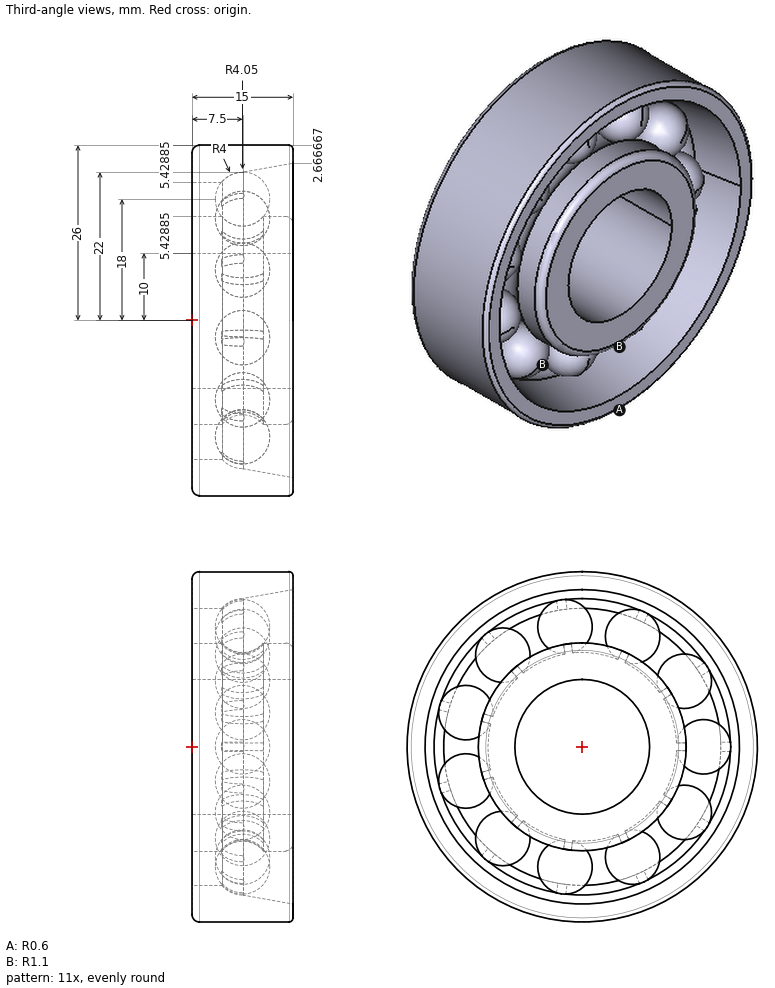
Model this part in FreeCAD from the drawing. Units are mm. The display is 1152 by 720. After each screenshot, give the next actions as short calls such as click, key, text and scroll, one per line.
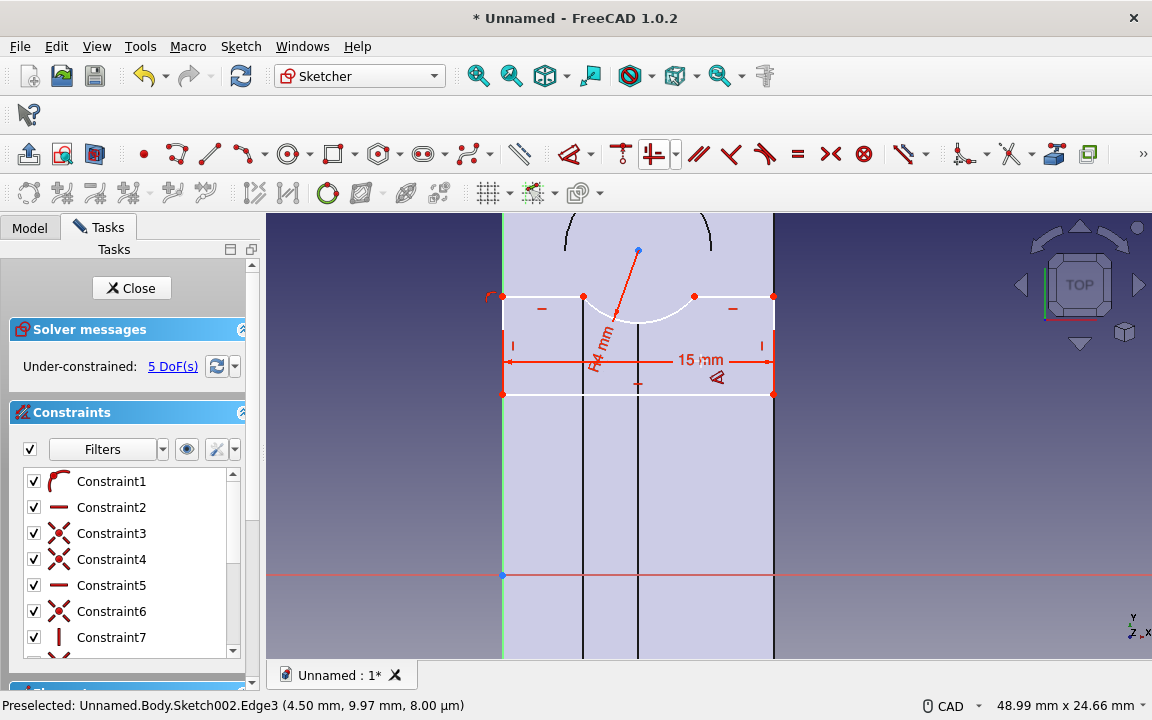
click(503, 395)
click(469, 485)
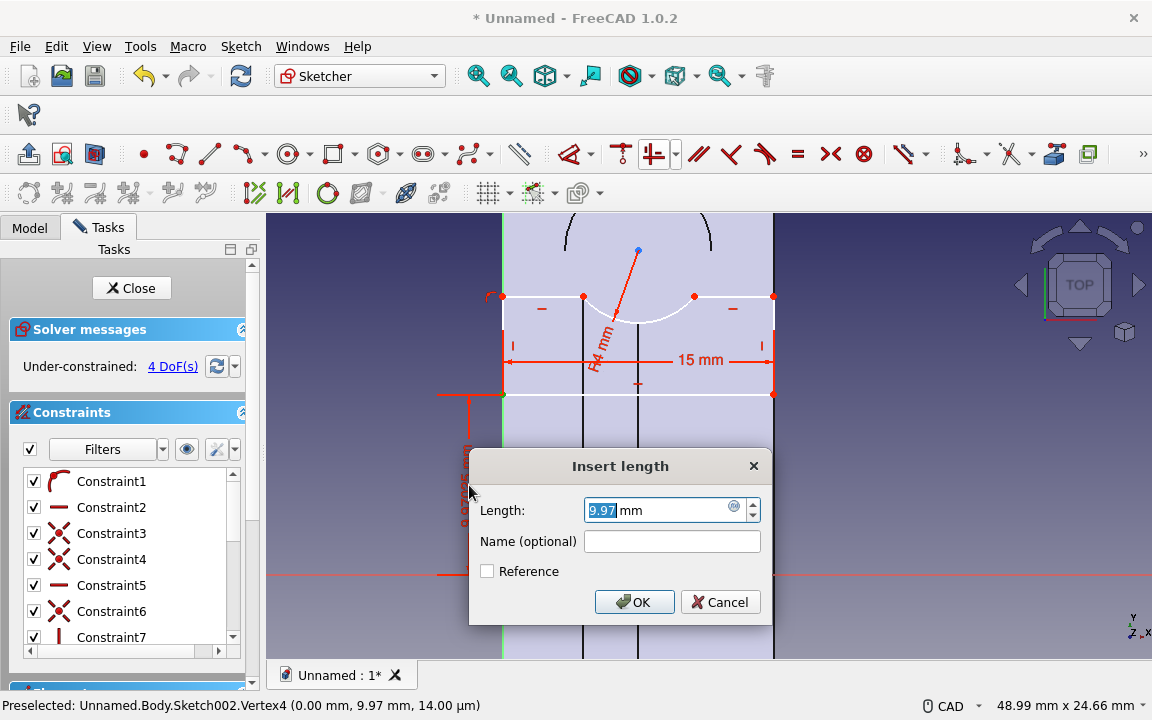
text(10)
key(Return)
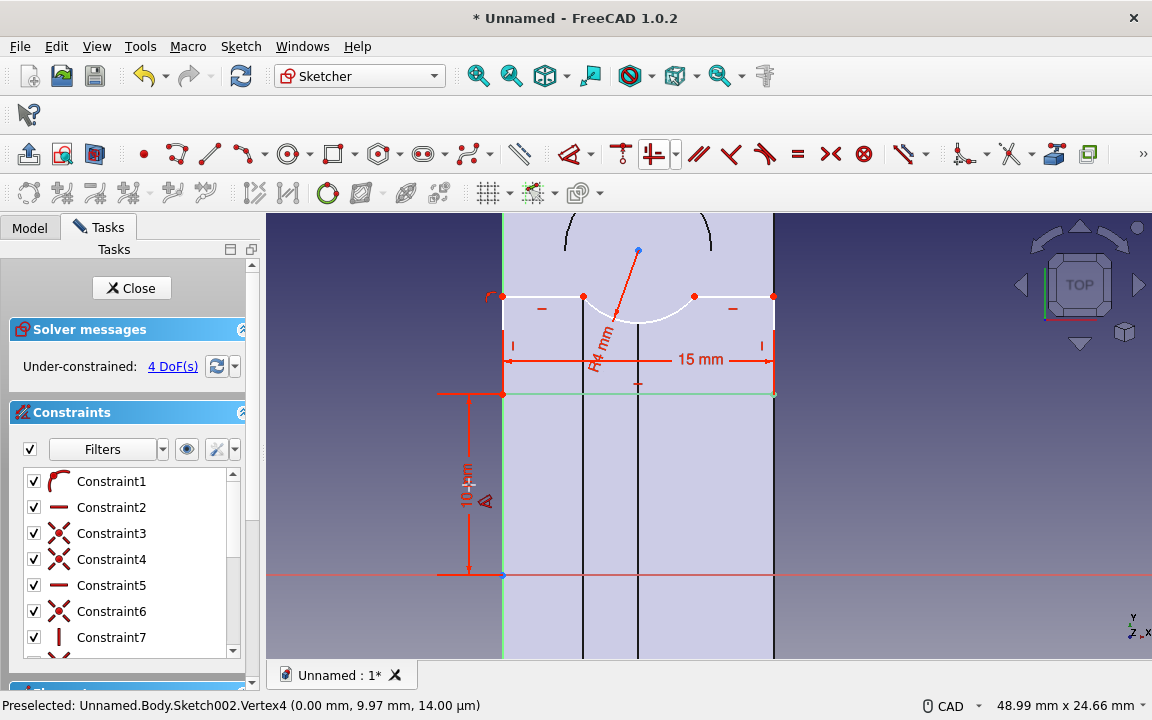
click(638, 251)
click(469, 413)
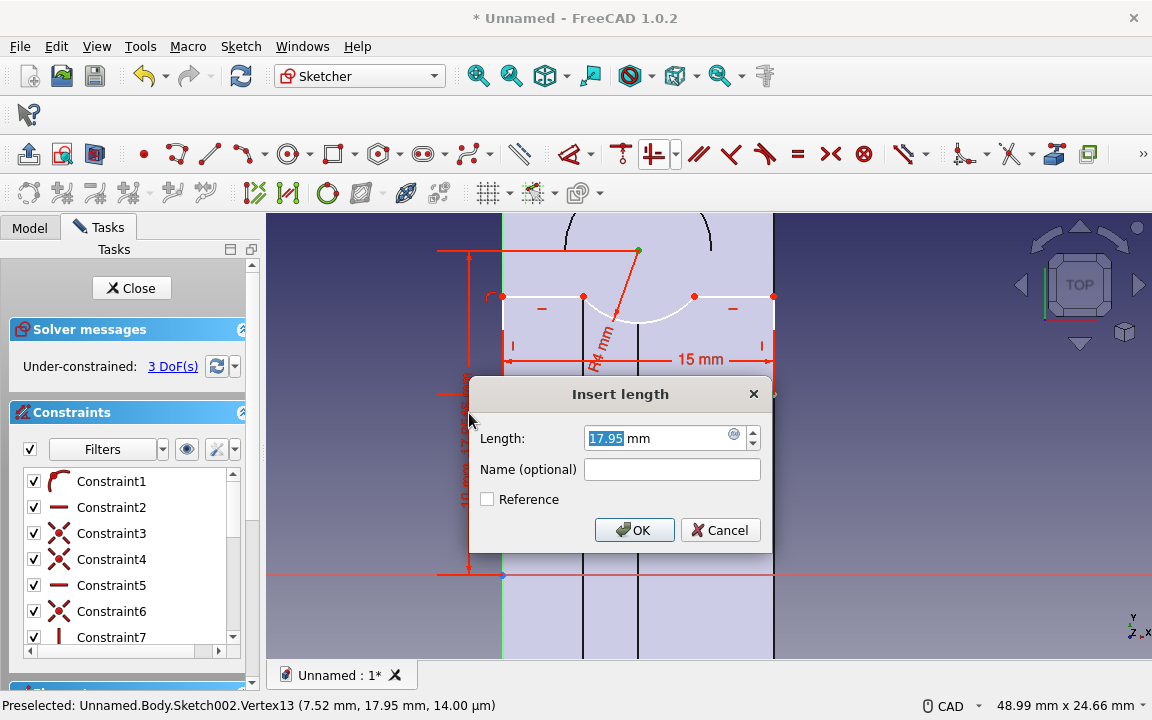
text(18)
key(Return)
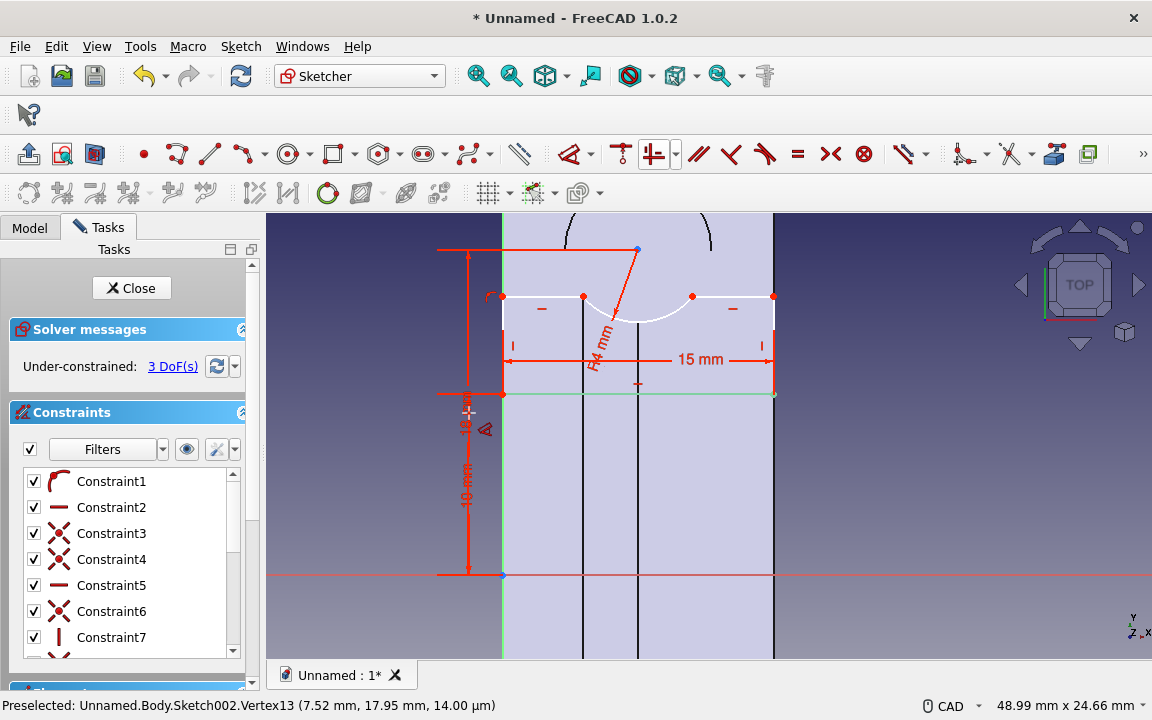
click(638, 250)
click(570, 609)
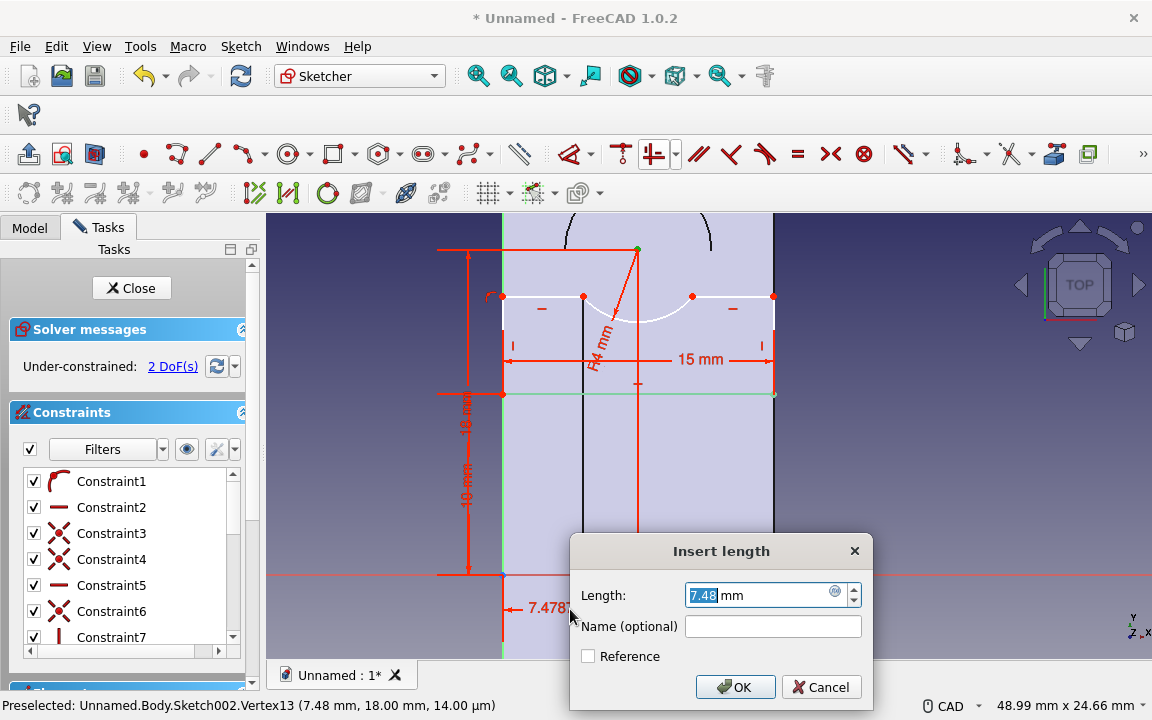
text(7.5)
key(Return)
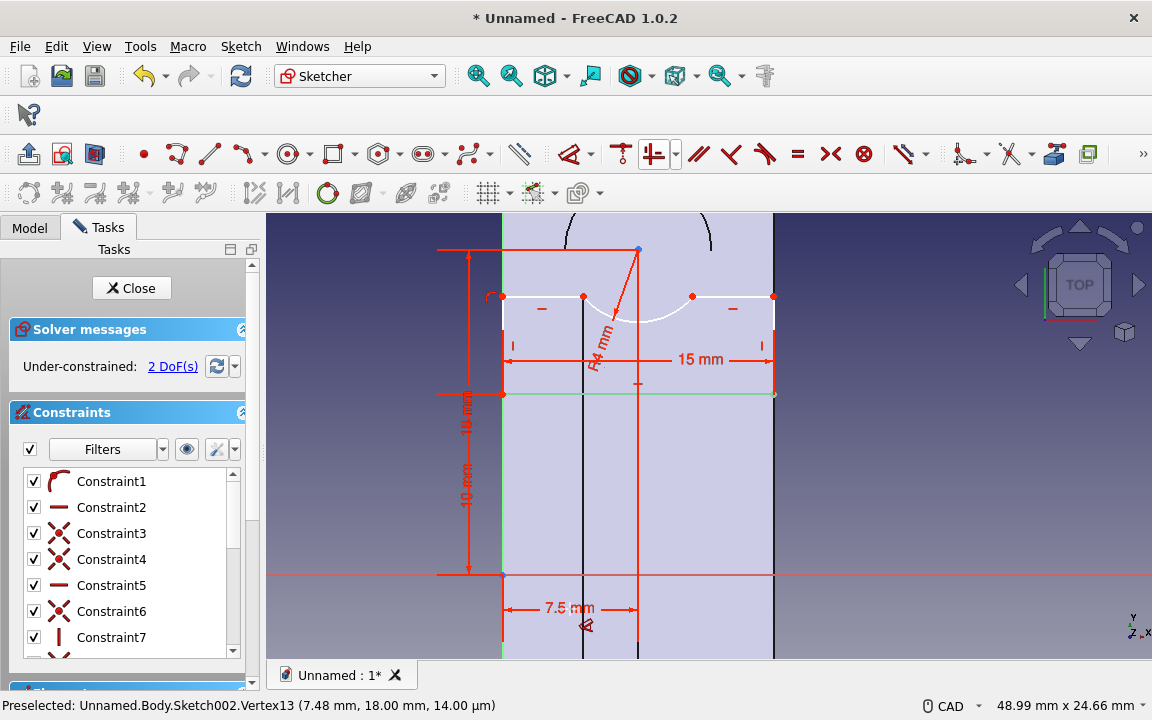
click(503, 326)
click(469, 346)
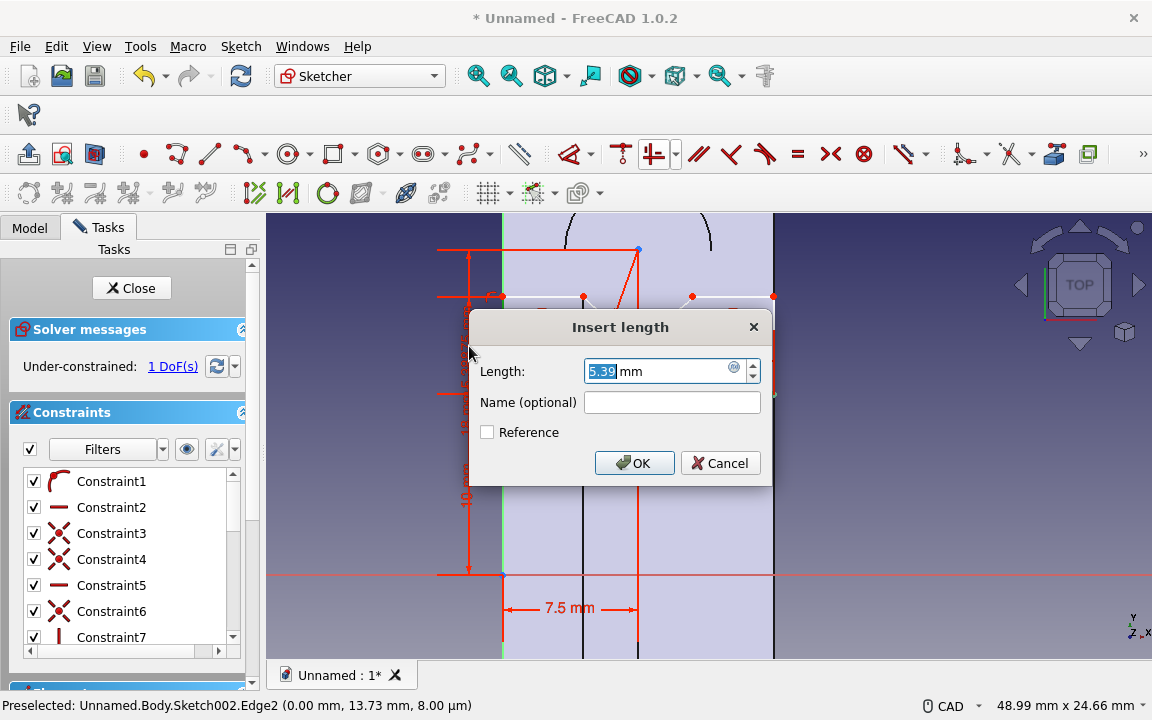
text(5.42885)
key(Return)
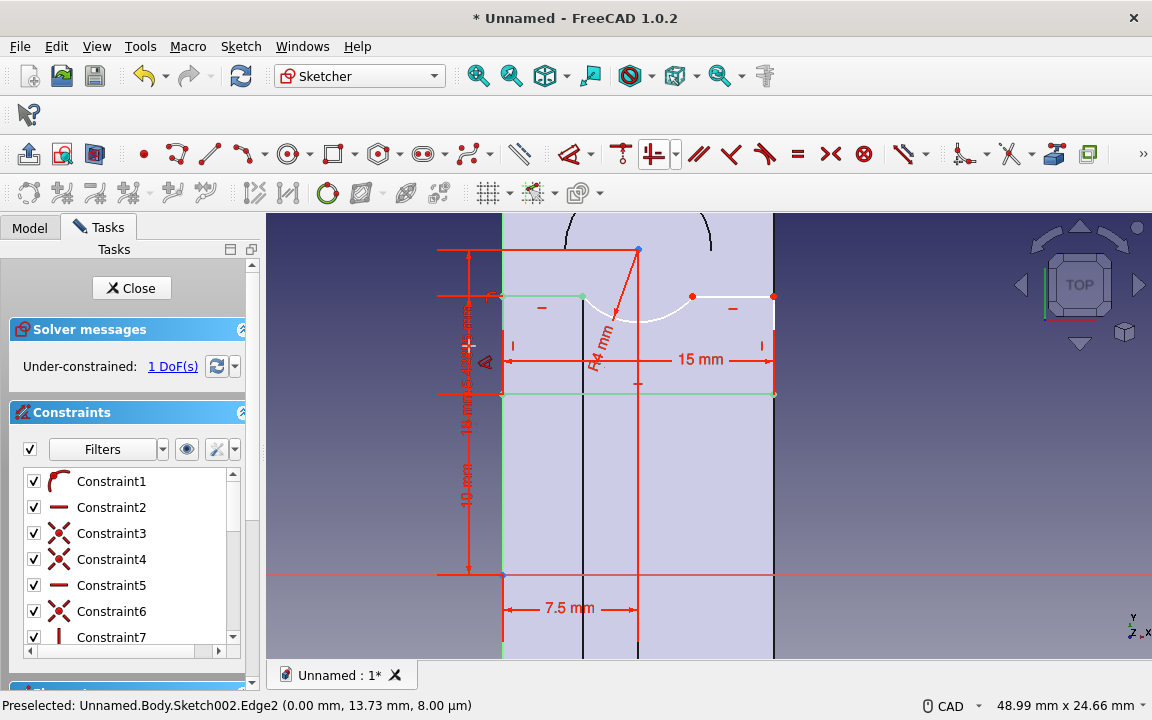
click(774, 365)
click(808, 346)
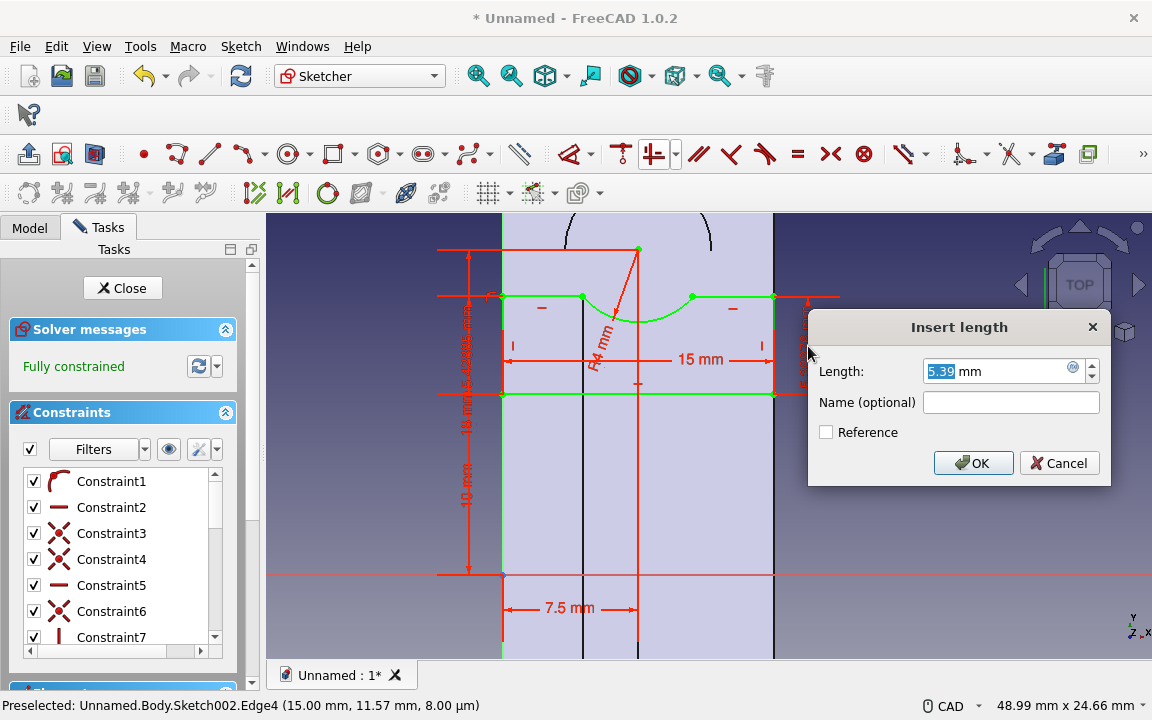
text(5.42885)
key(Return)
key(Escape)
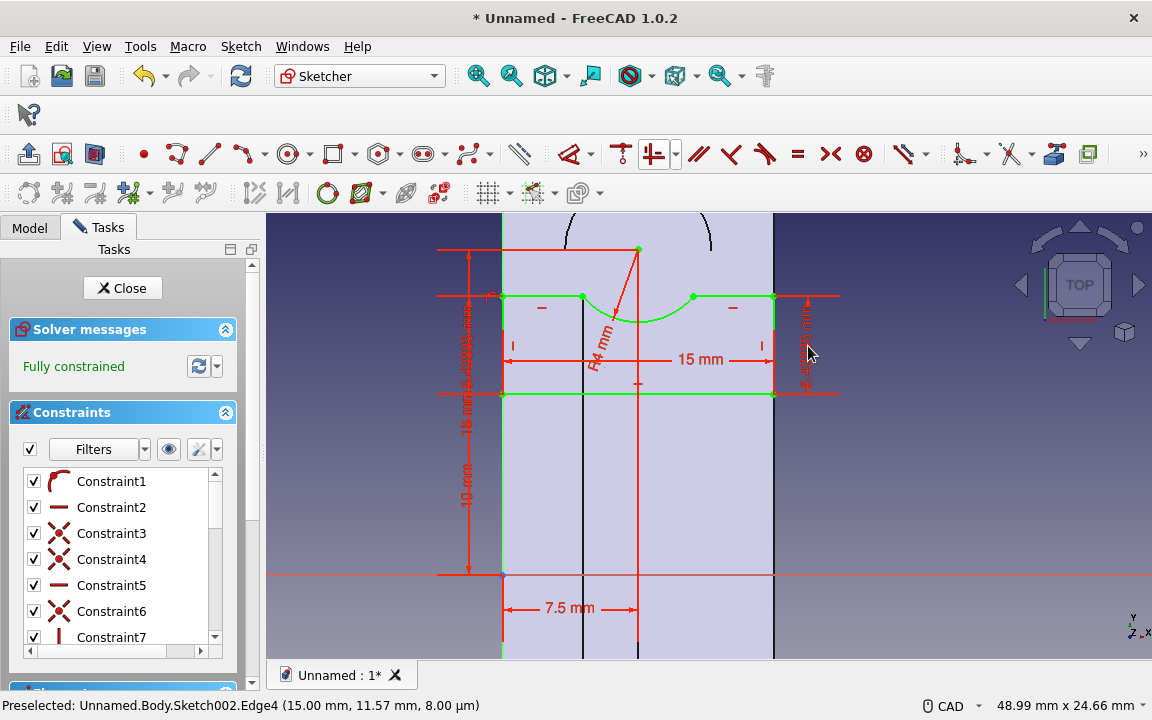
click(123, 288)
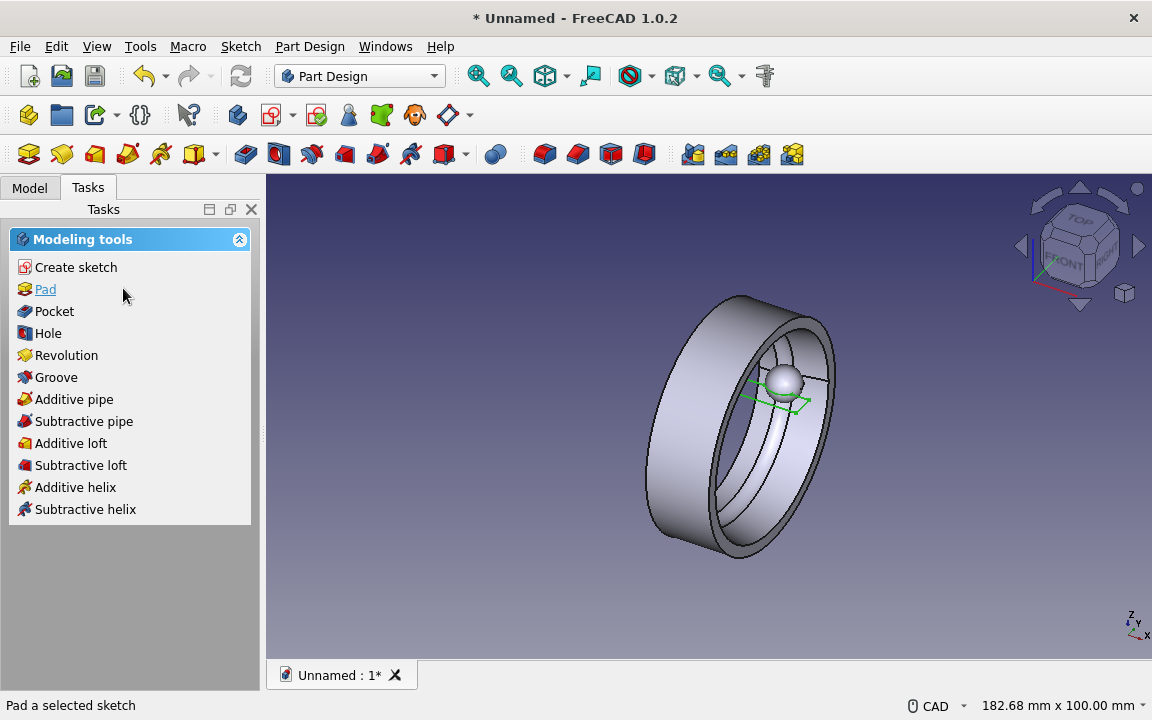
click(62, 154)